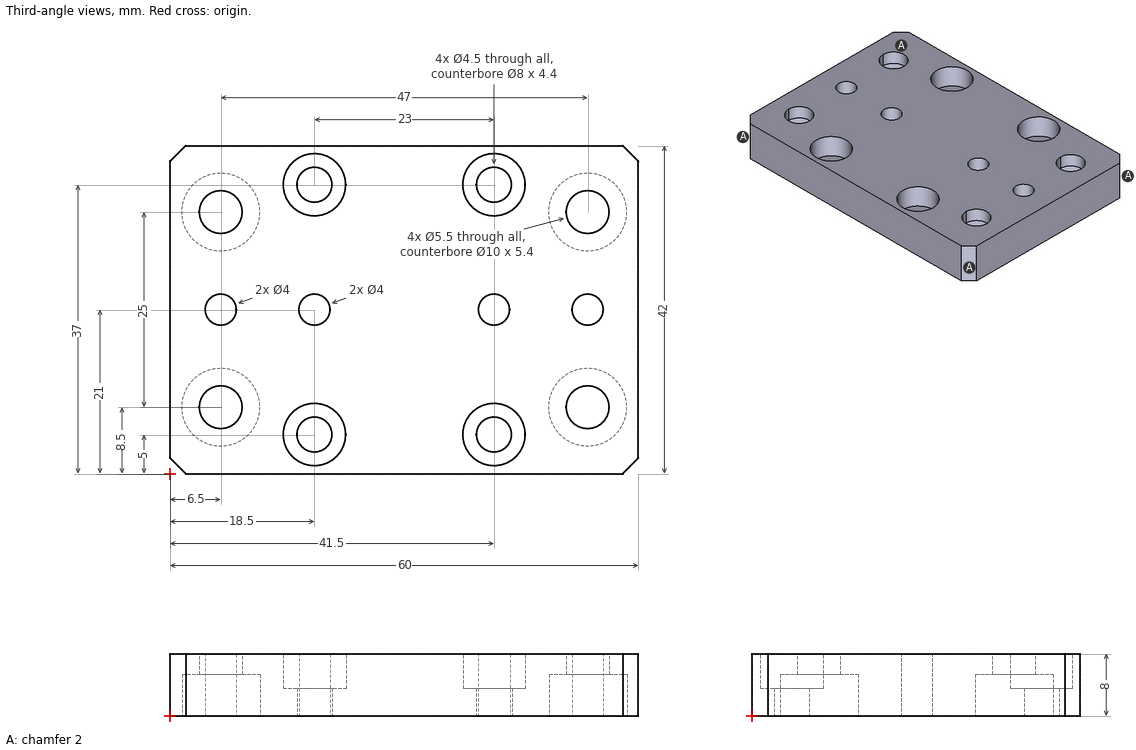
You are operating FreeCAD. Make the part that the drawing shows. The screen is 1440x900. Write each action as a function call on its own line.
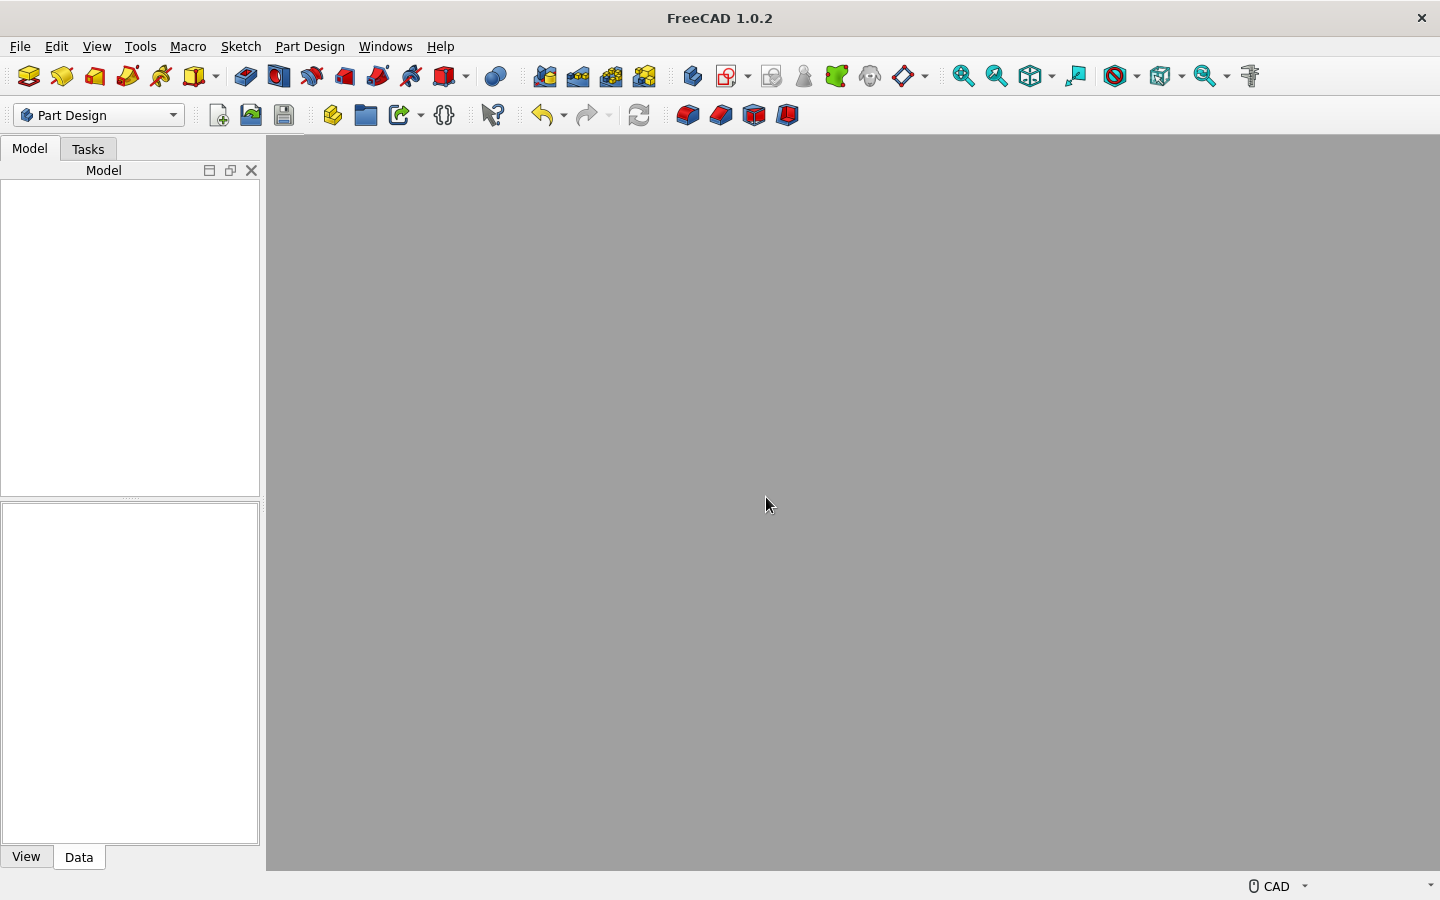
key(ctrl+n)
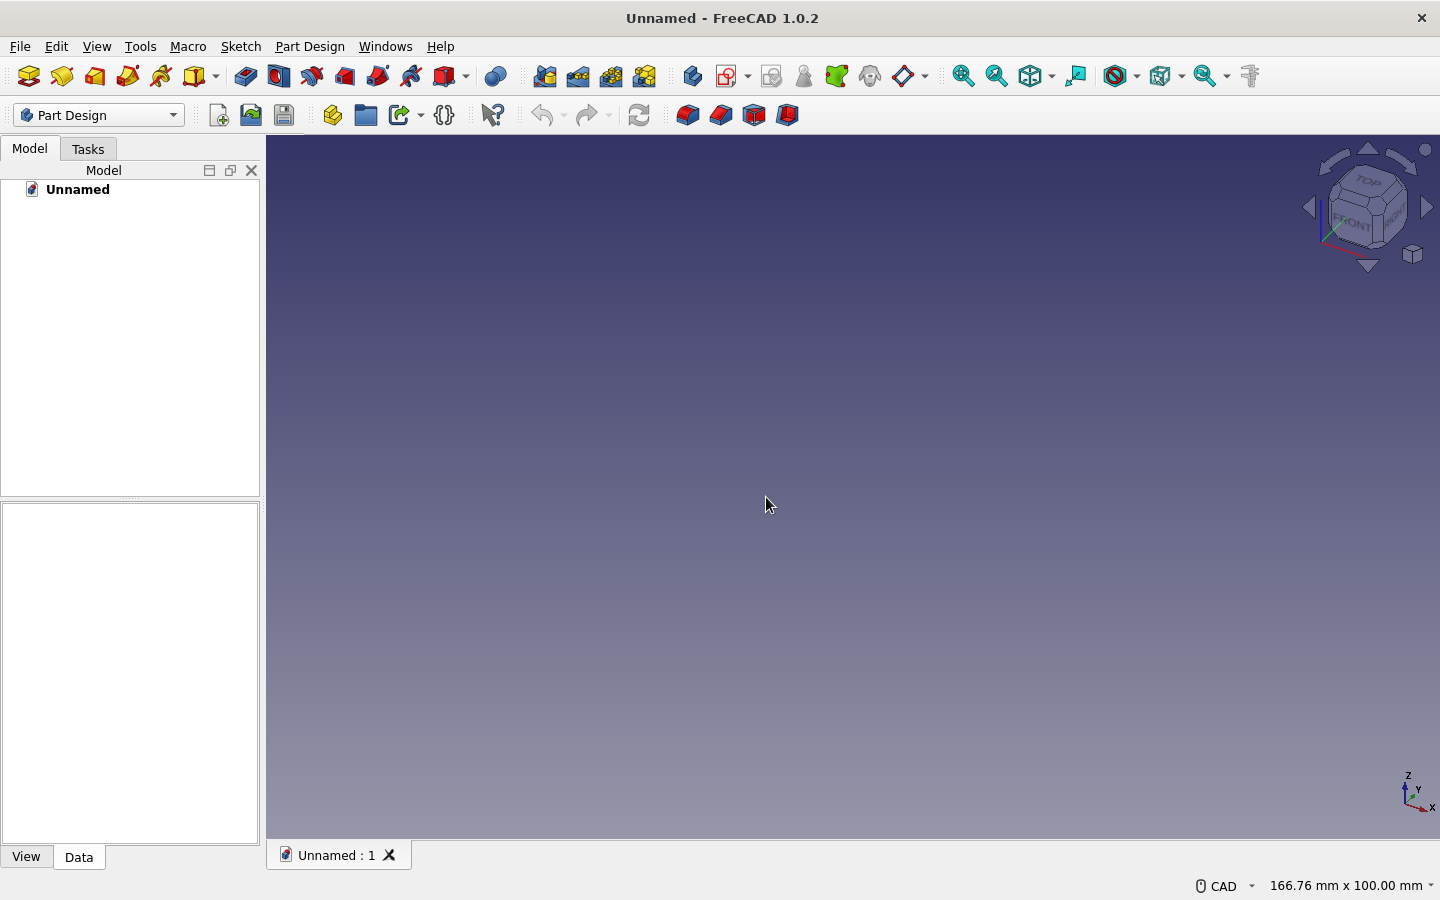
click(726, 76)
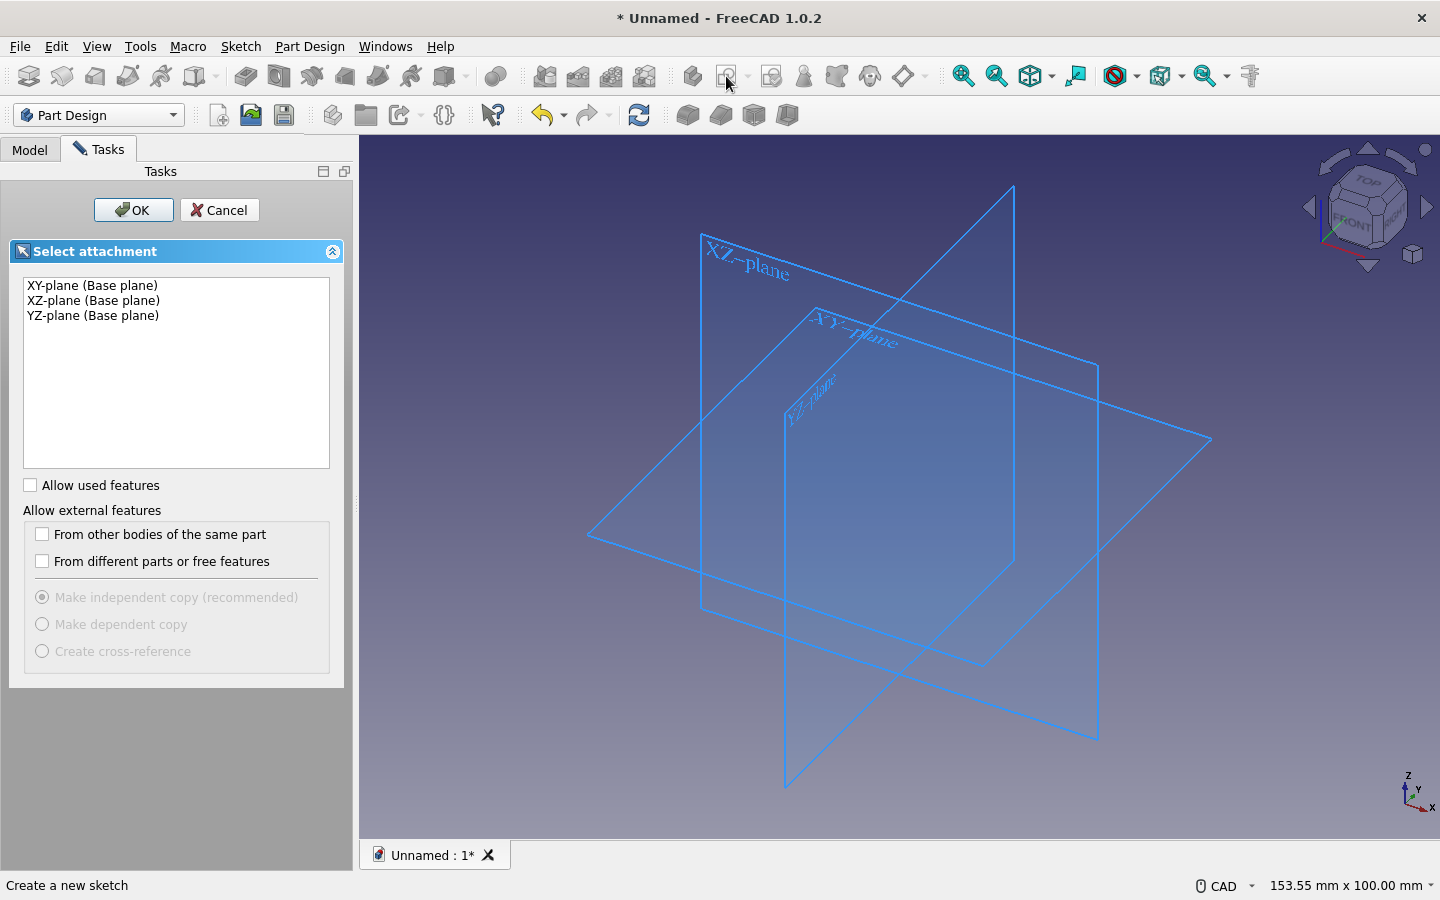
click(84, 286)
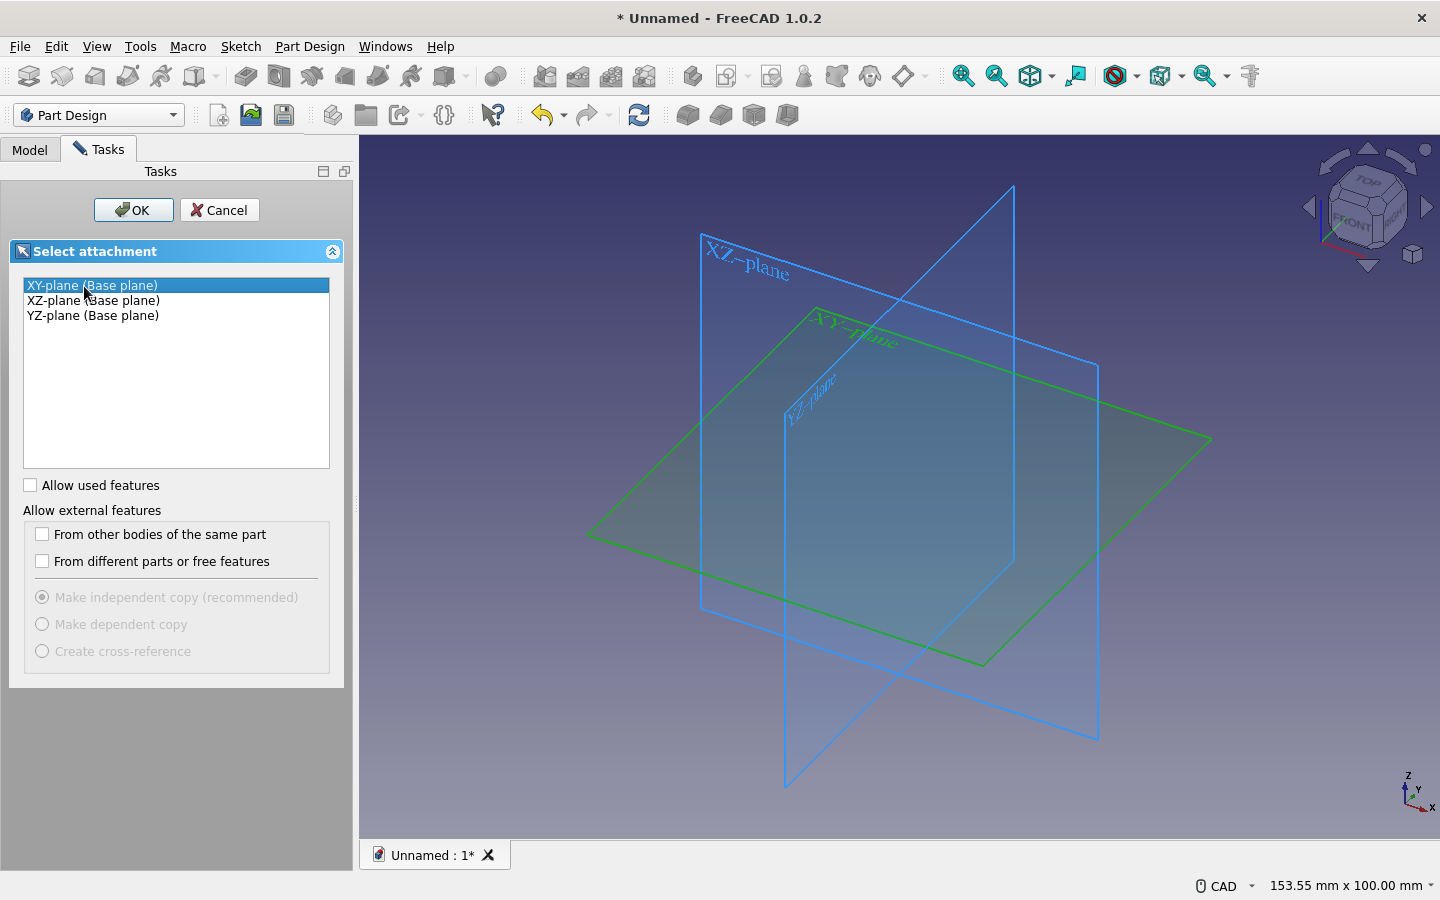
click(134, 210)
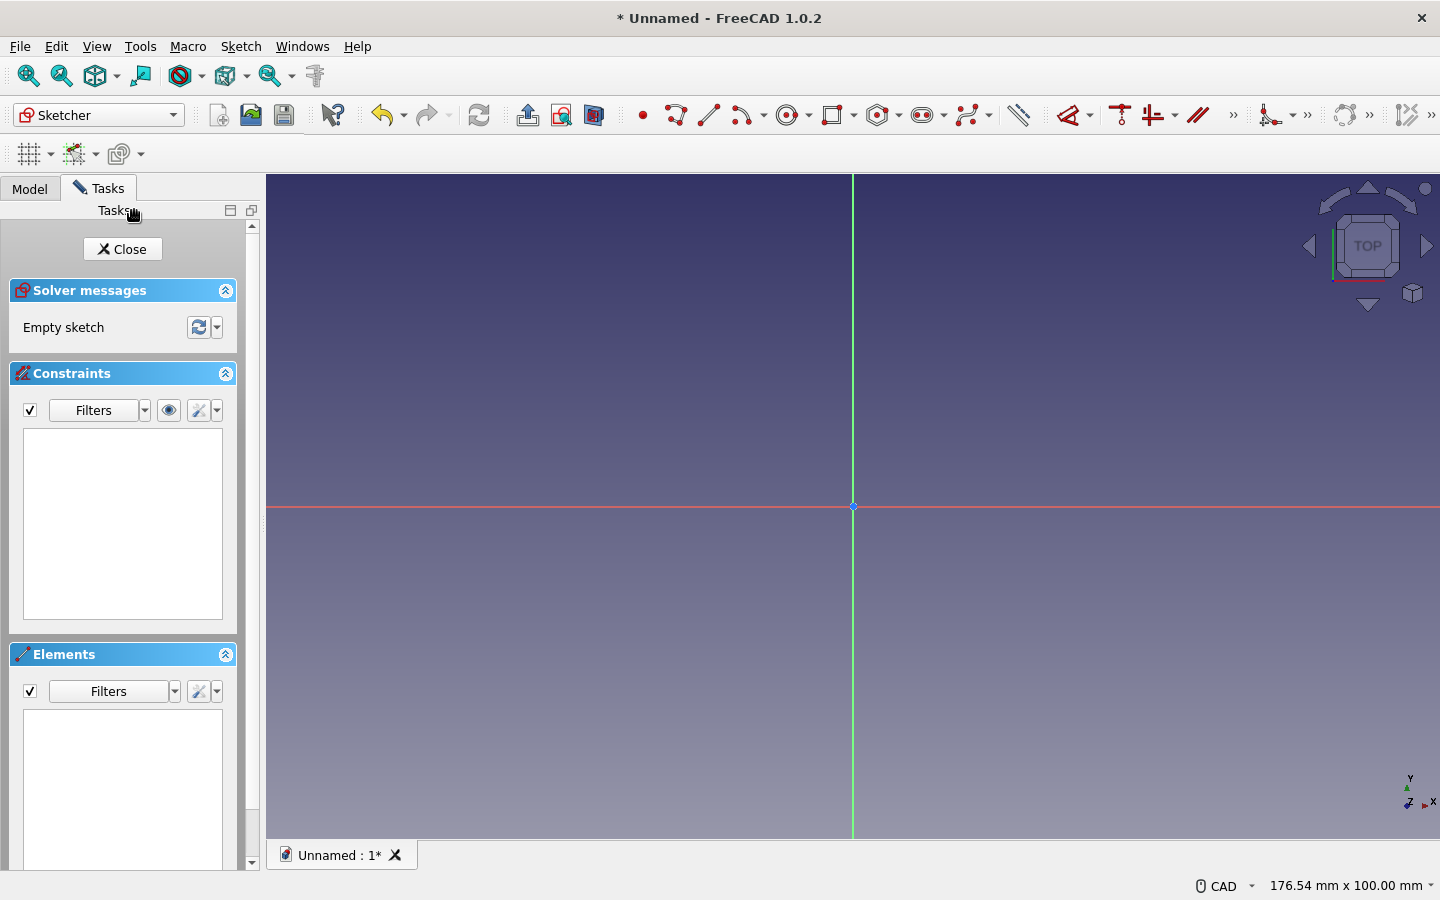
scroll(1275, 202, up, 2)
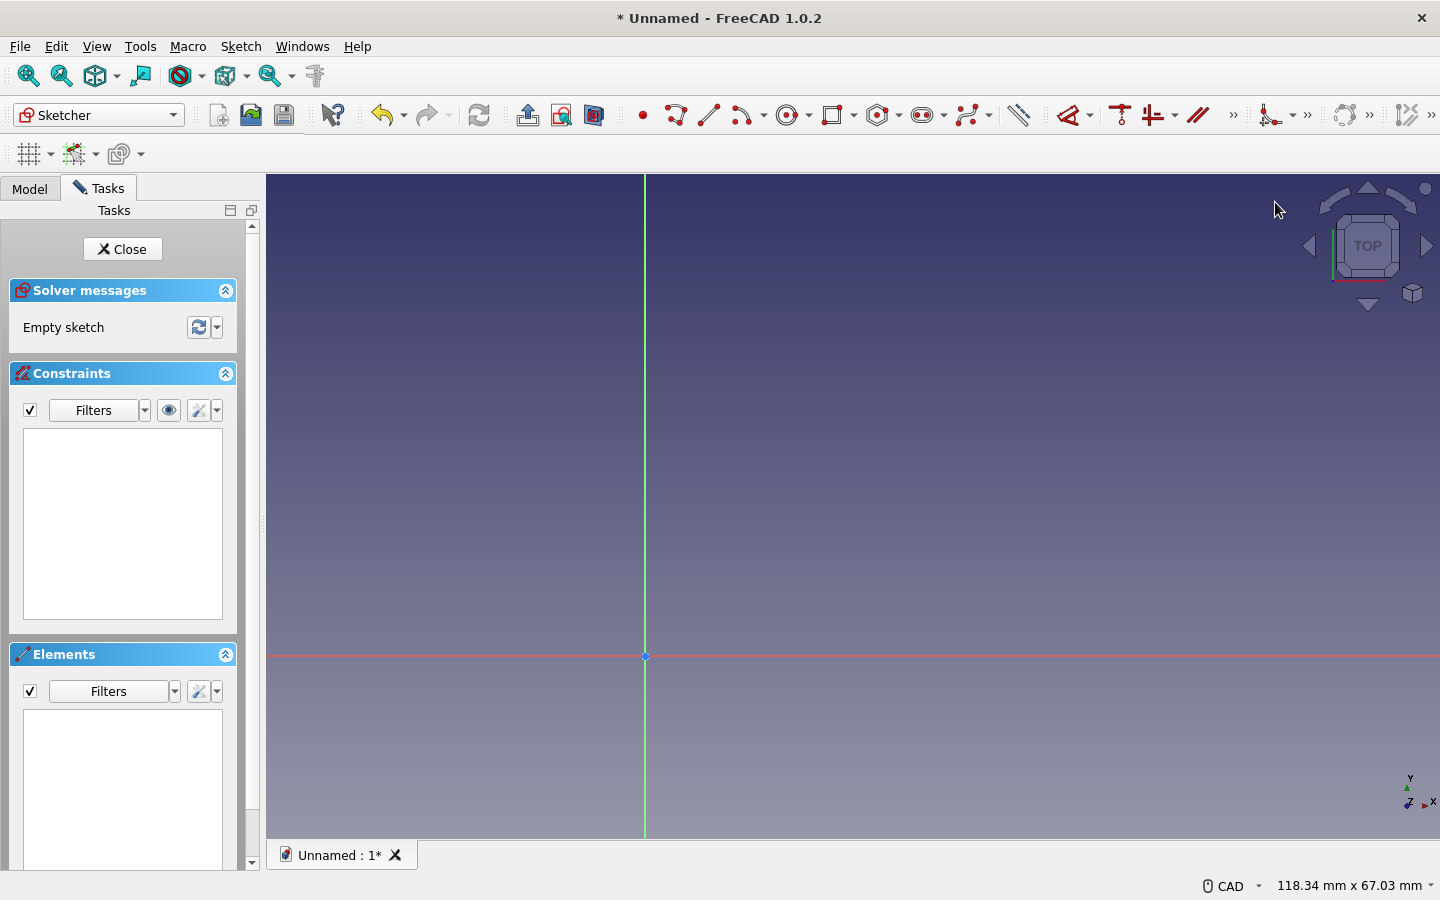
click(832, 116)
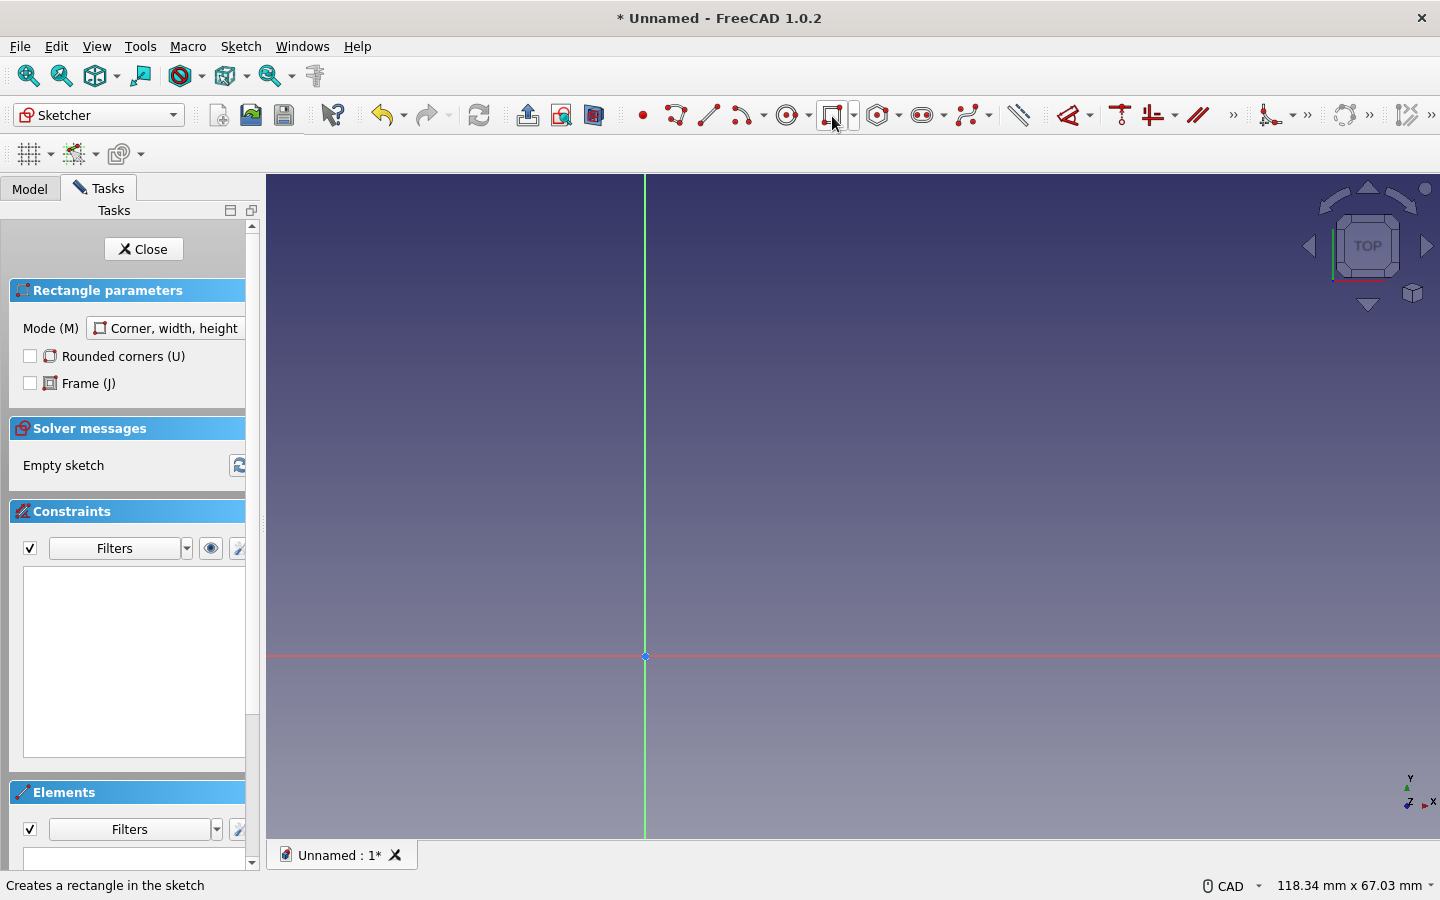
click(645, 656)
click(1240, 240)
key(Escape)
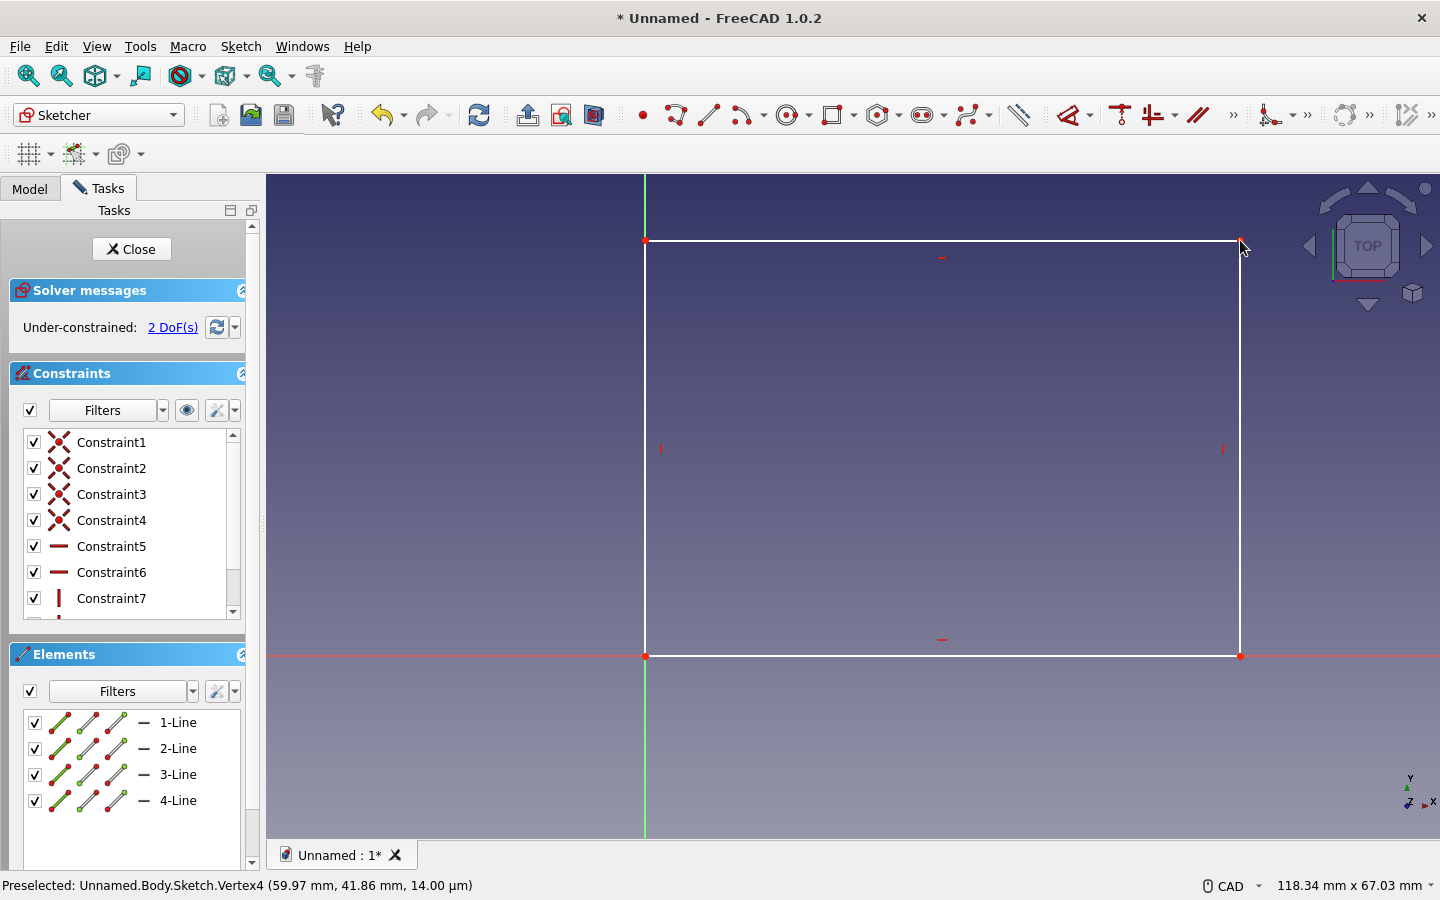
click(824, 656)